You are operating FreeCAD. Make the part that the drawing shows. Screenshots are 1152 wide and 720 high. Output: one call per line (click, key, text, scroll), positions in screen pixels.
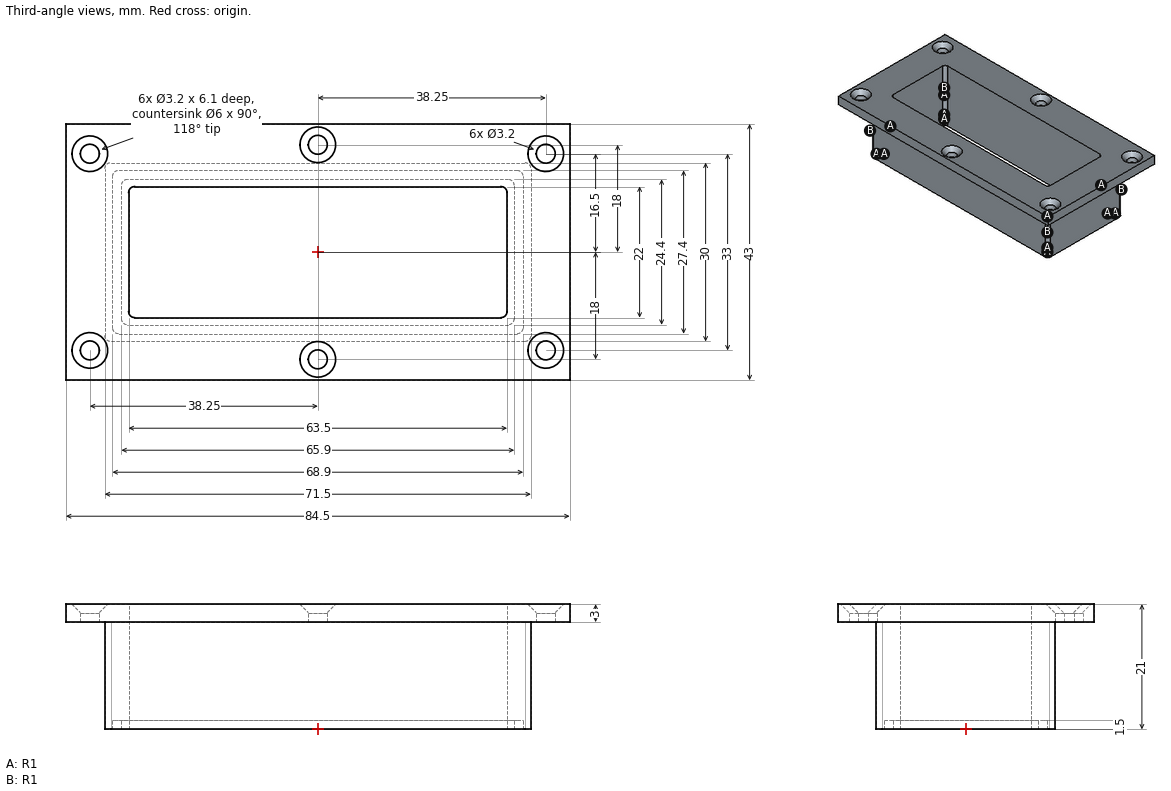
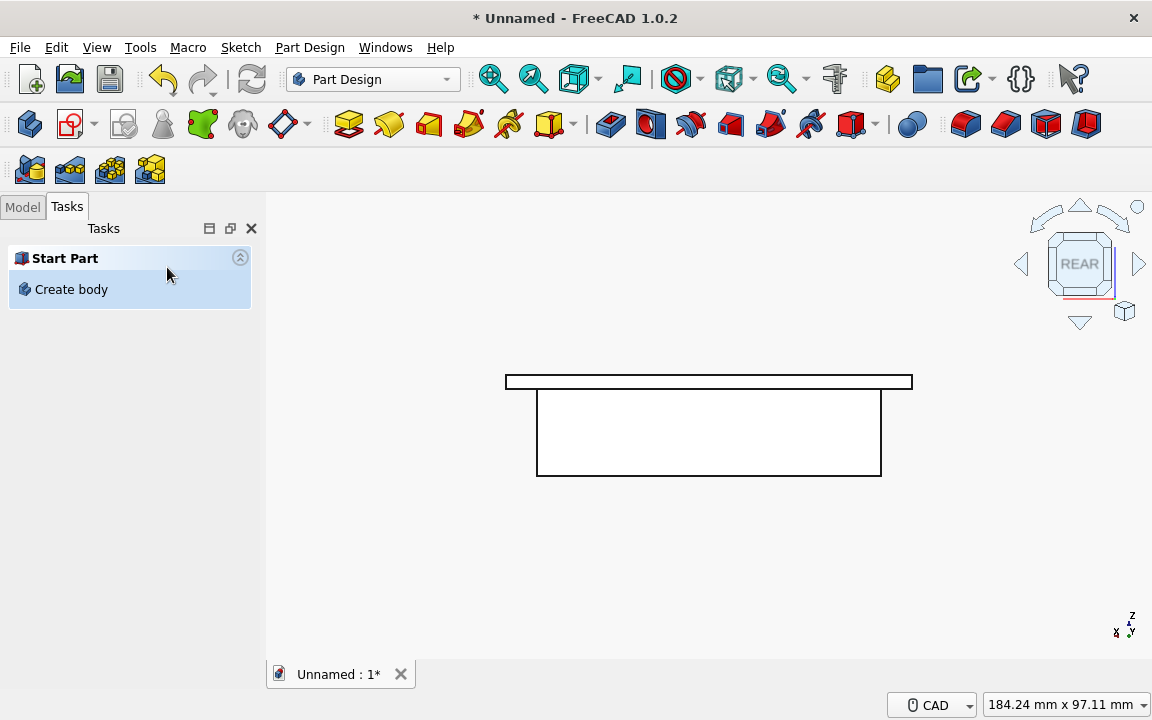
key(6)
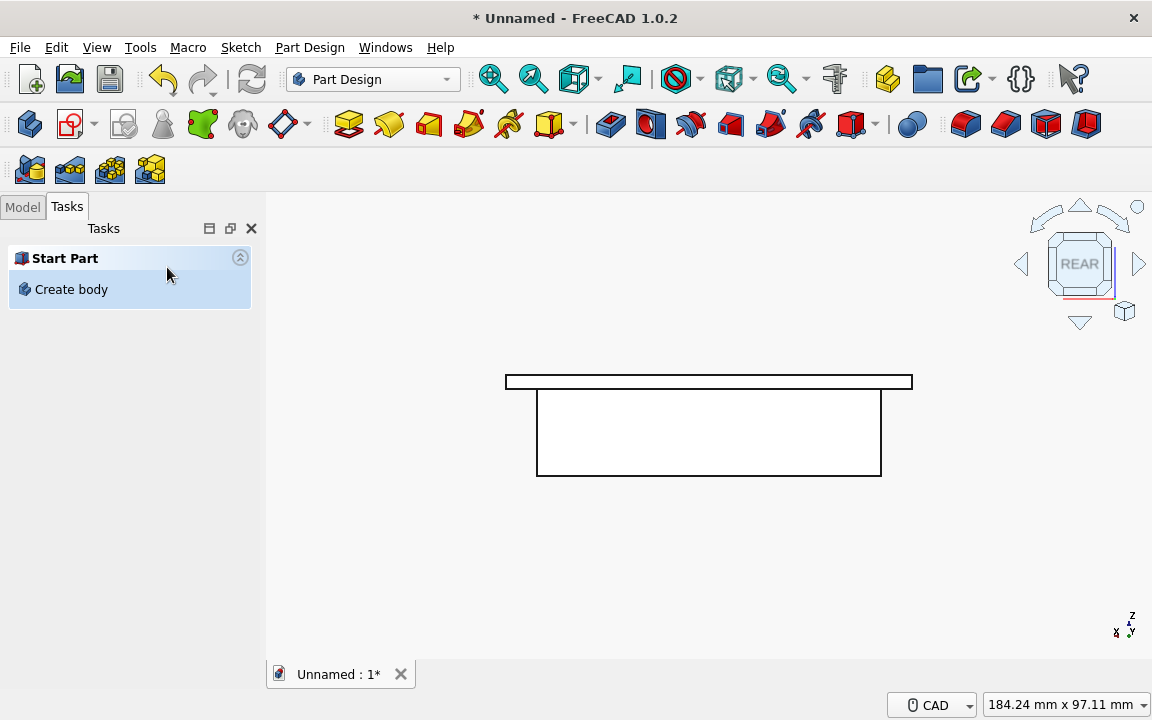
click(494, 80)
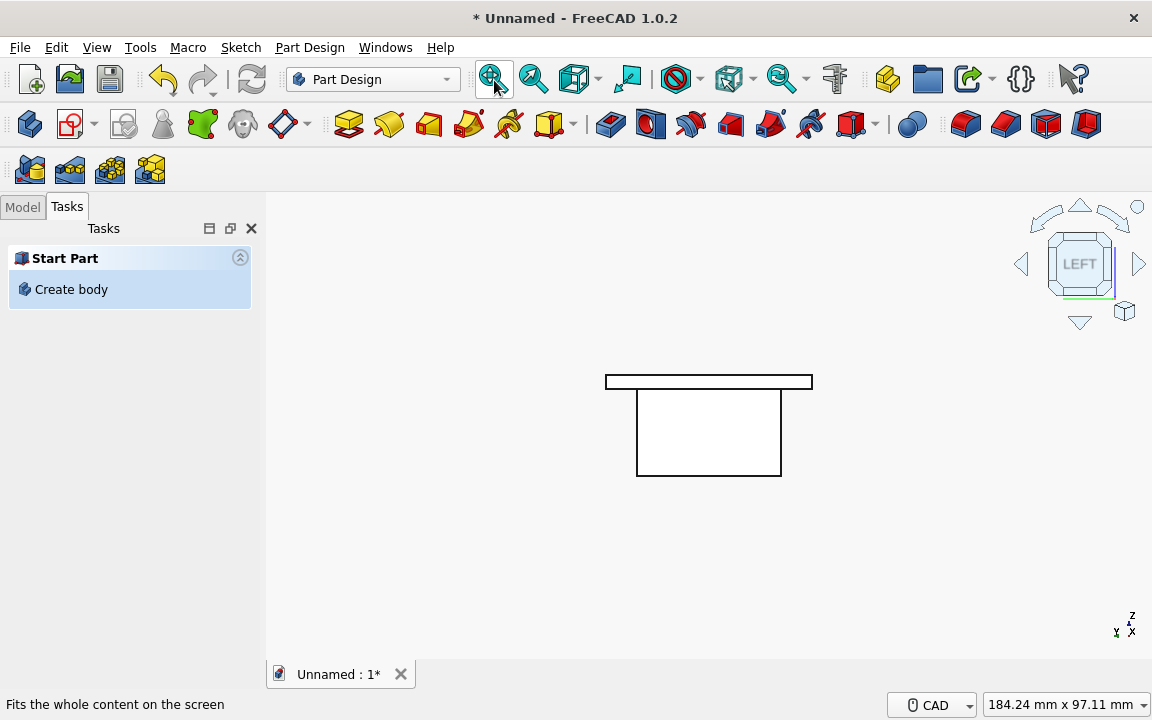
key(v)
key(3)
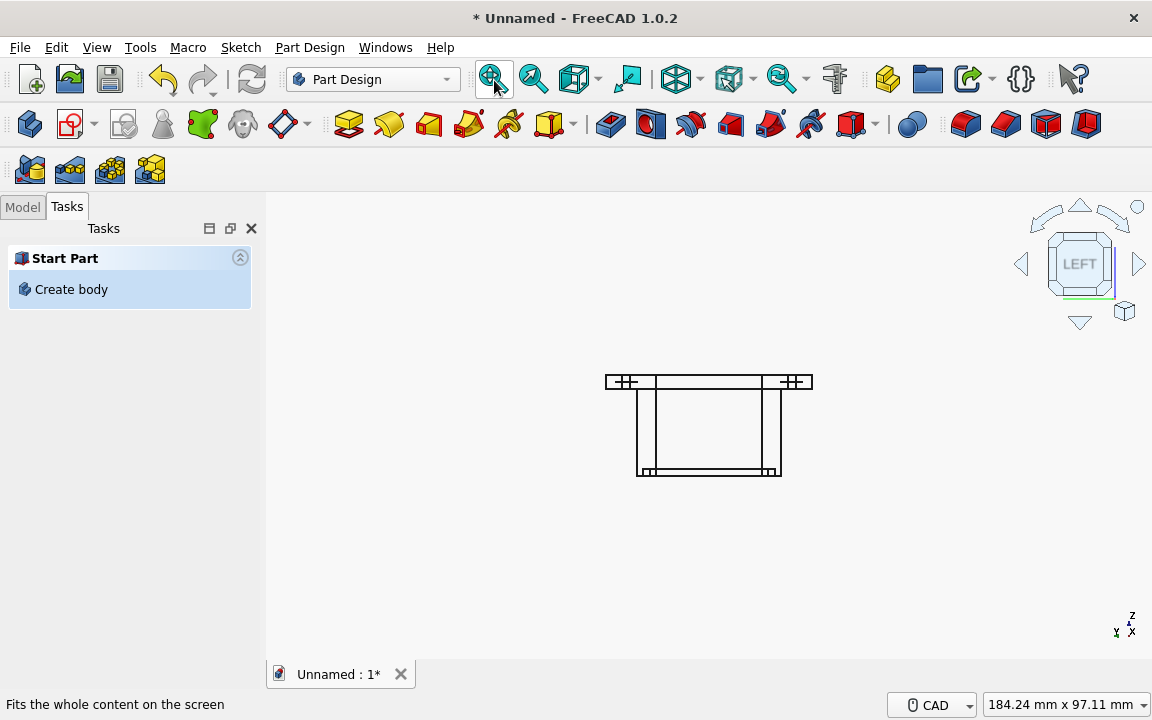
key(0)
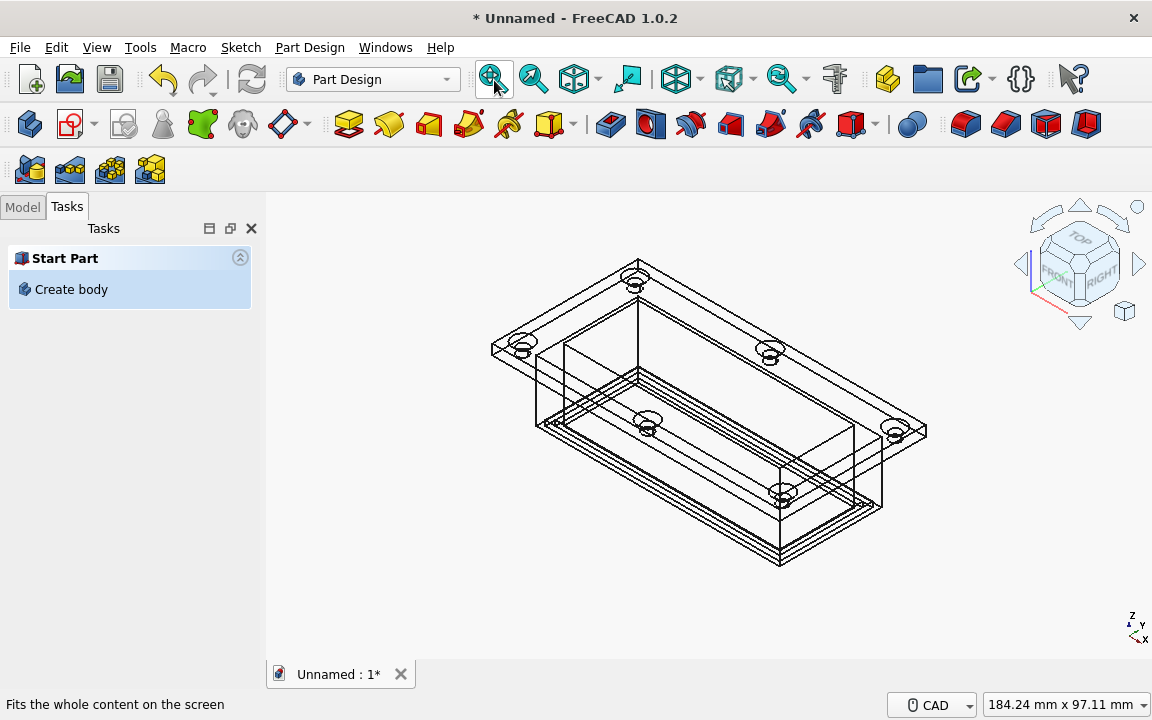
click(638, 341)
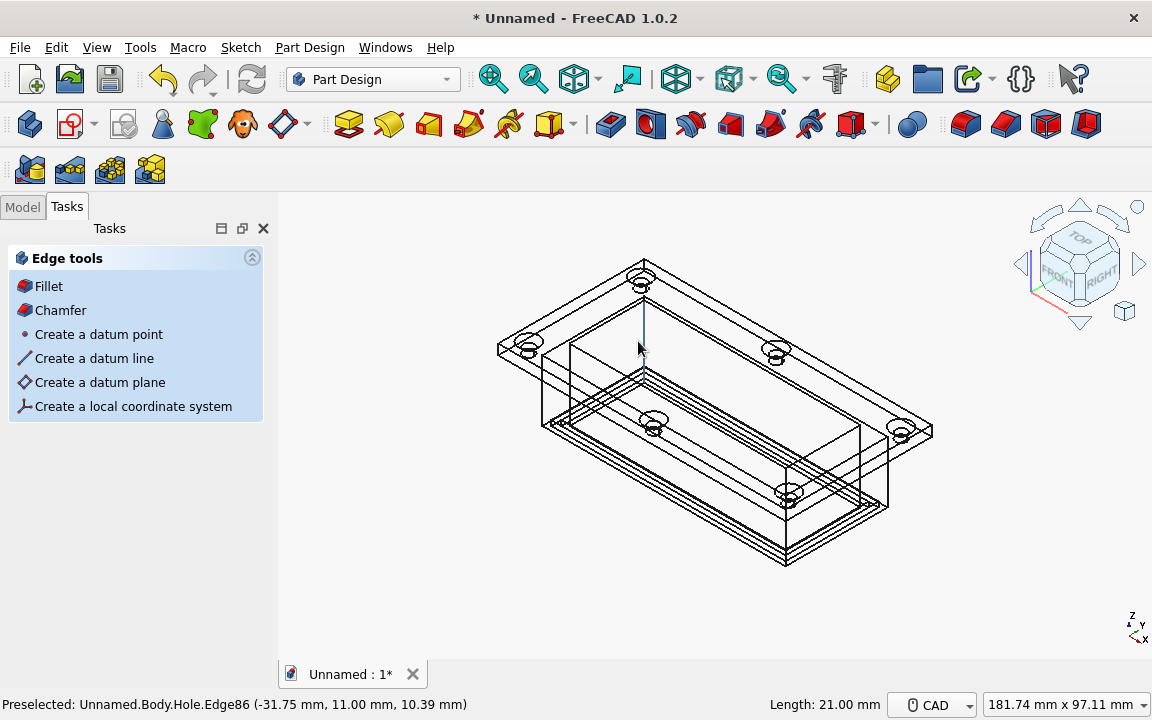
click(570, 408, ctrl)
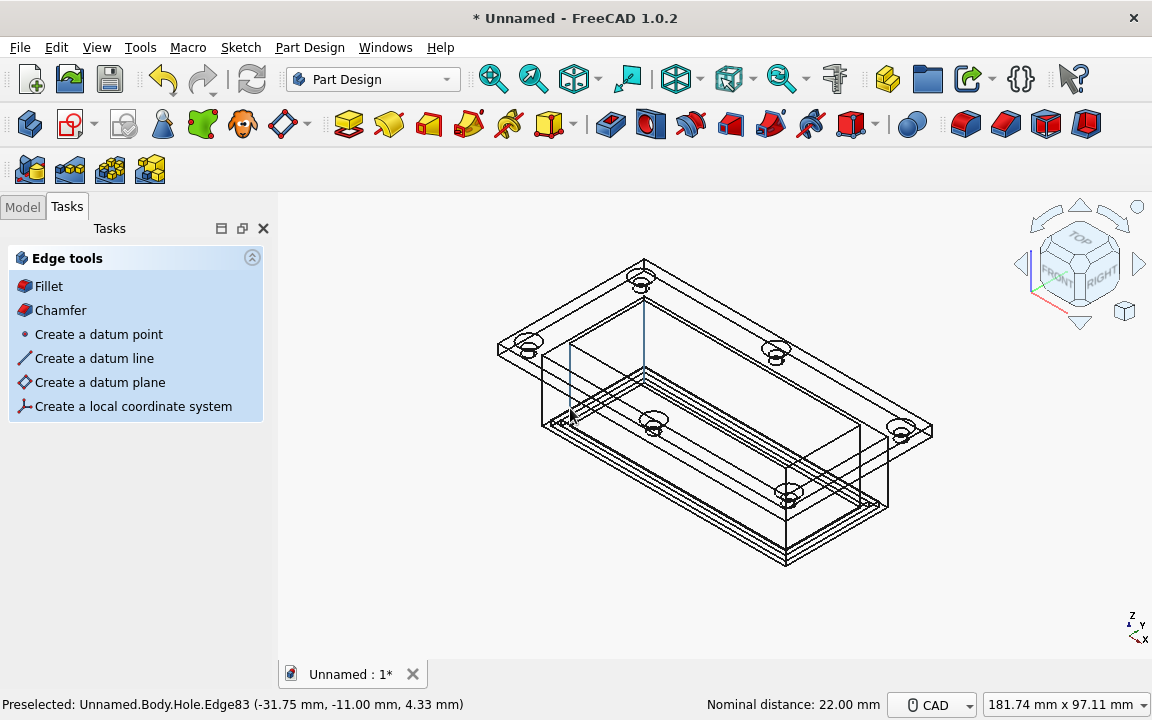
click(860, 490, ctrl)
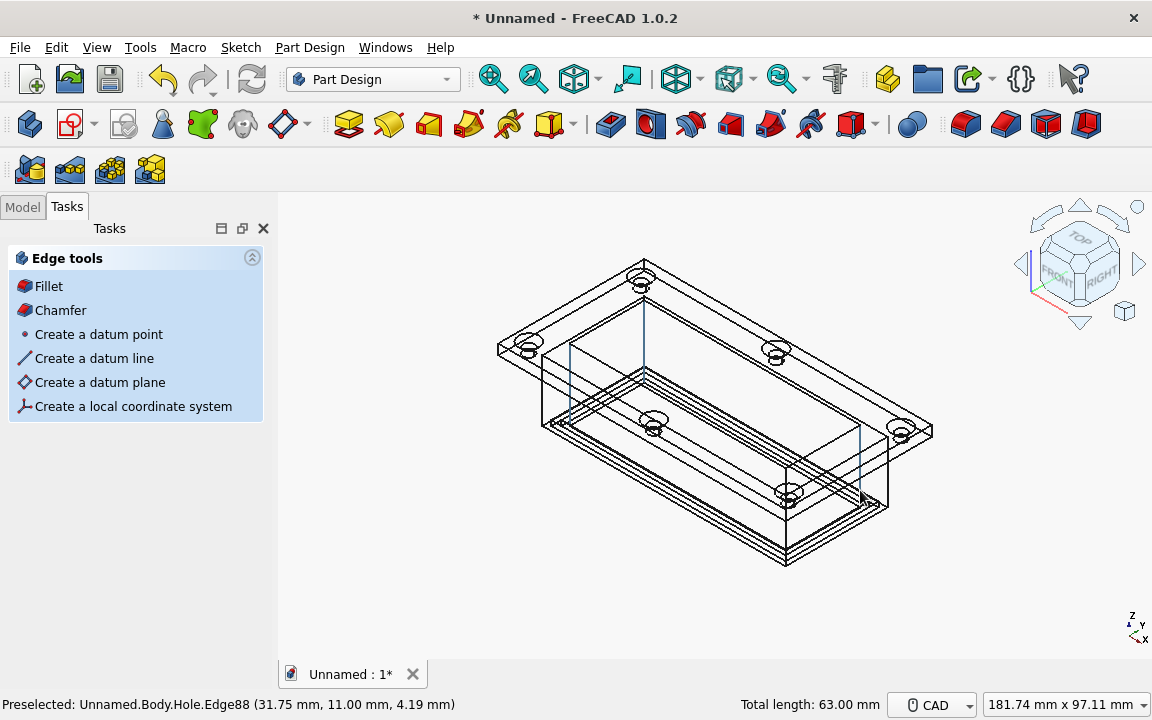
scroll(786, 508, up, 6)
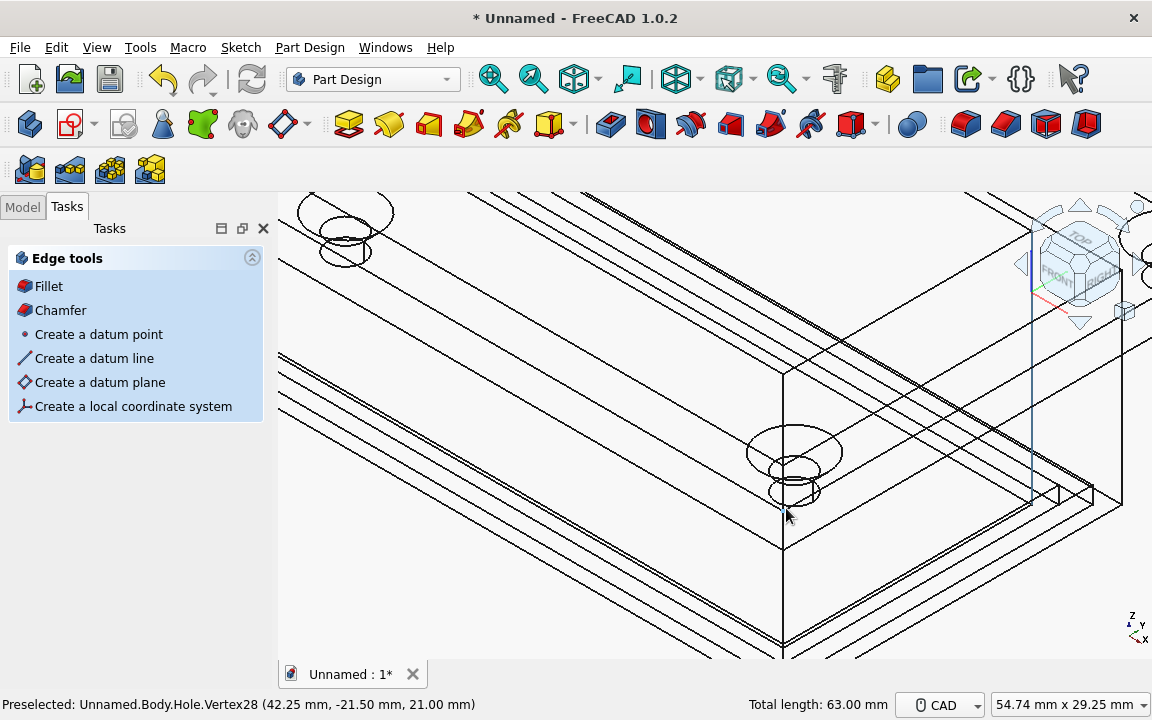
click(783, 406, ctrl)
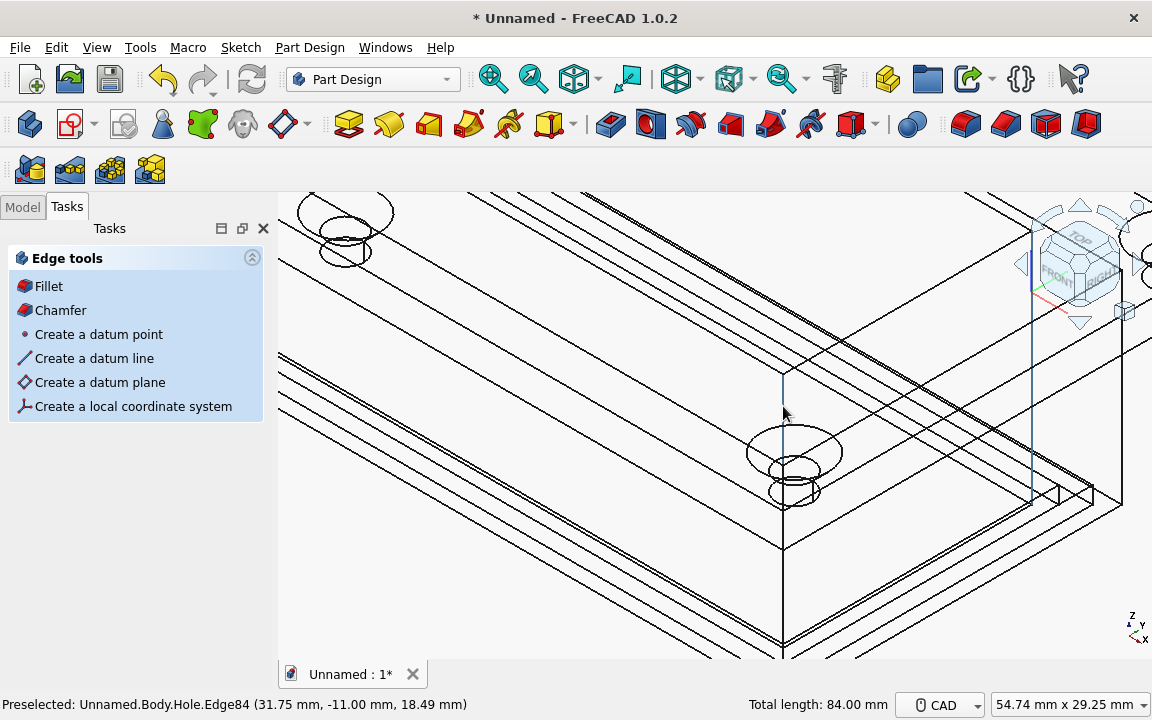
click(1059, 494, ctrl)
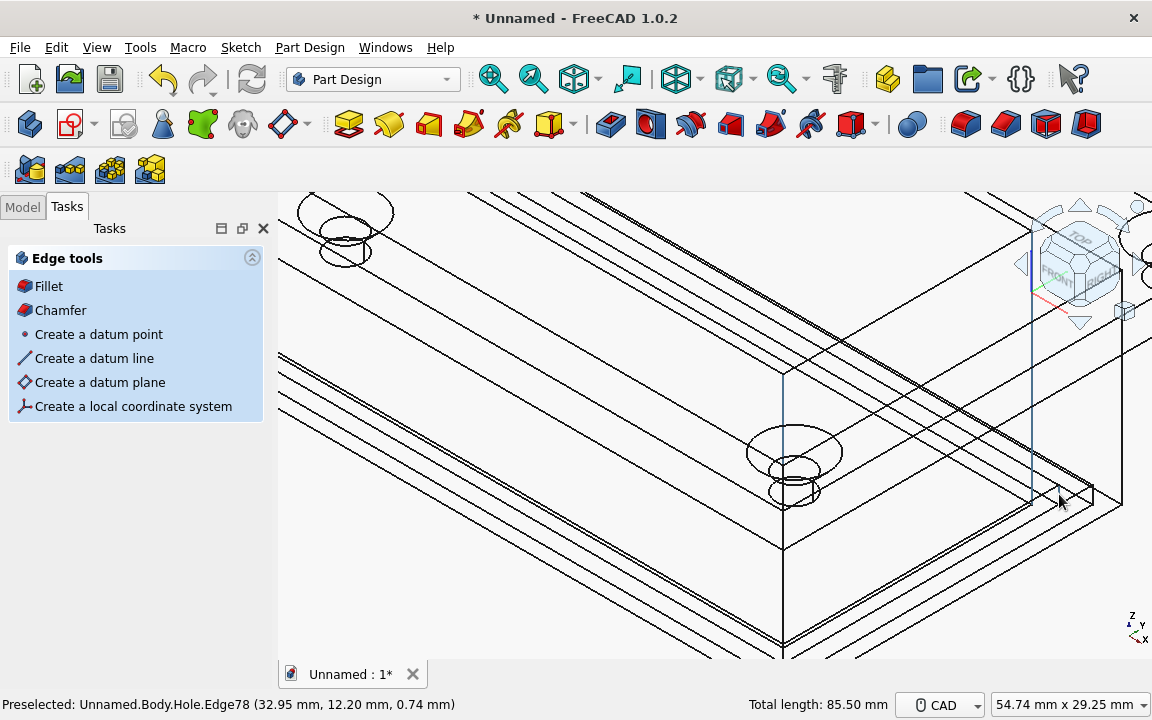
click(494, 80)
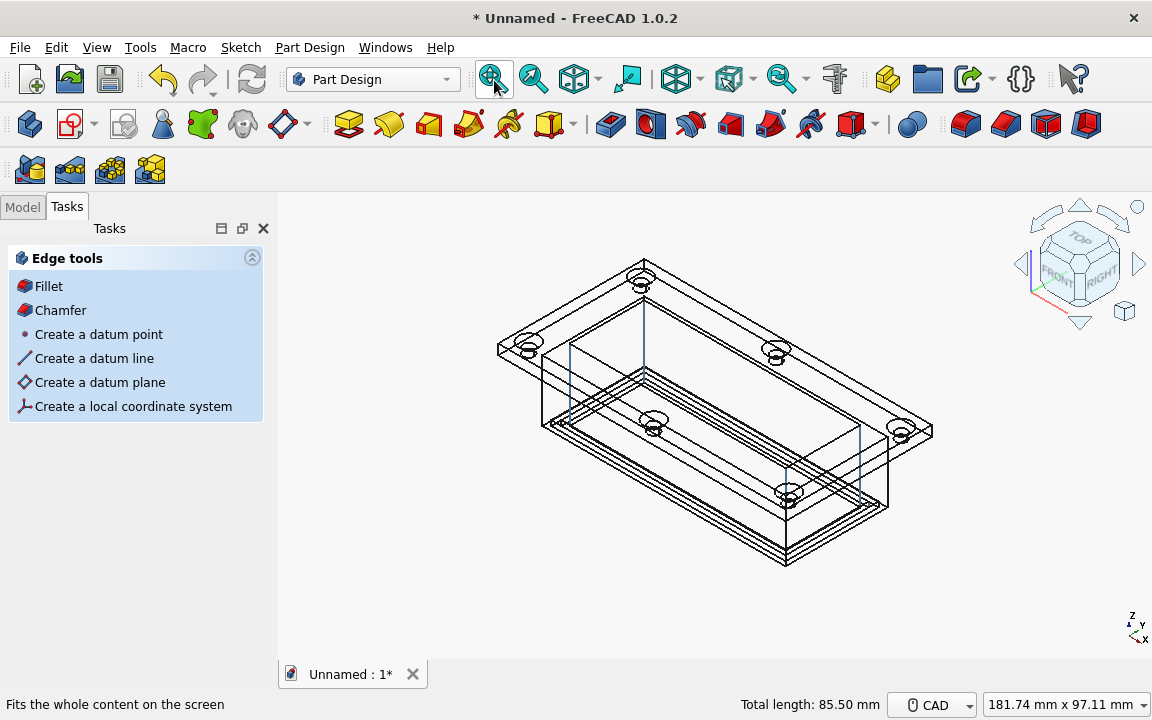
key(2)